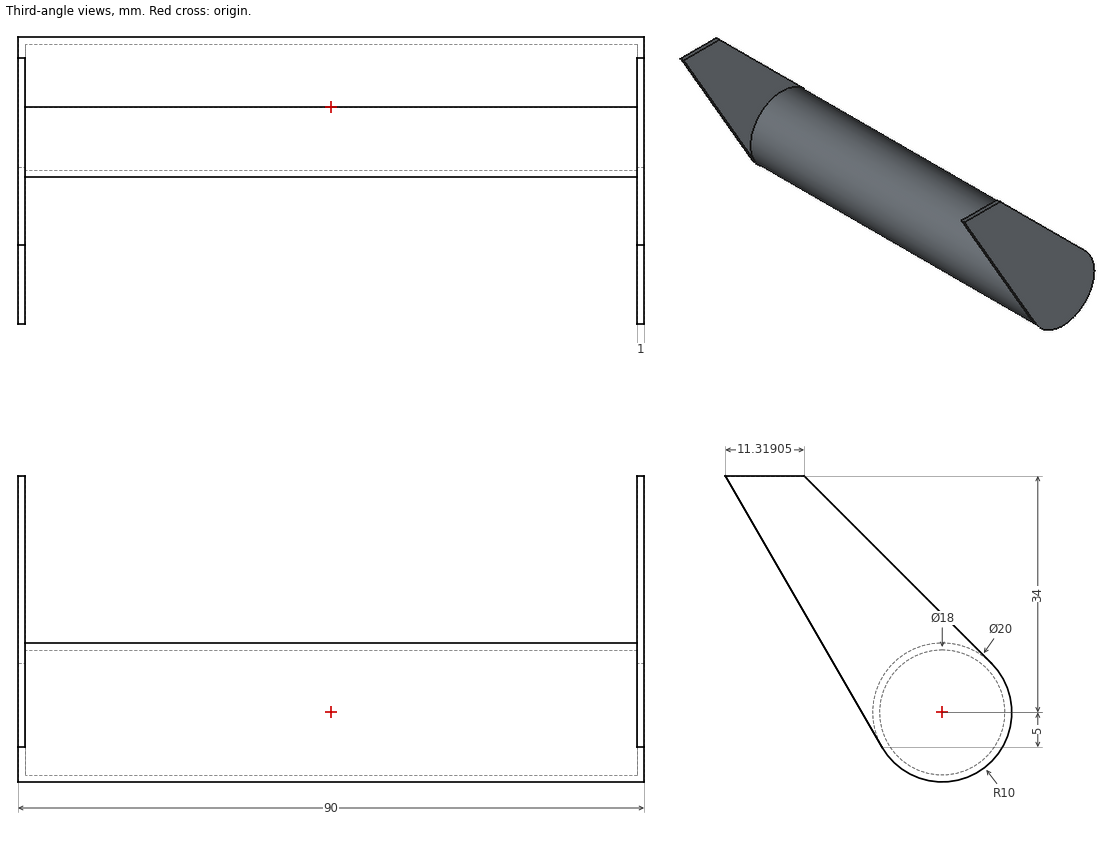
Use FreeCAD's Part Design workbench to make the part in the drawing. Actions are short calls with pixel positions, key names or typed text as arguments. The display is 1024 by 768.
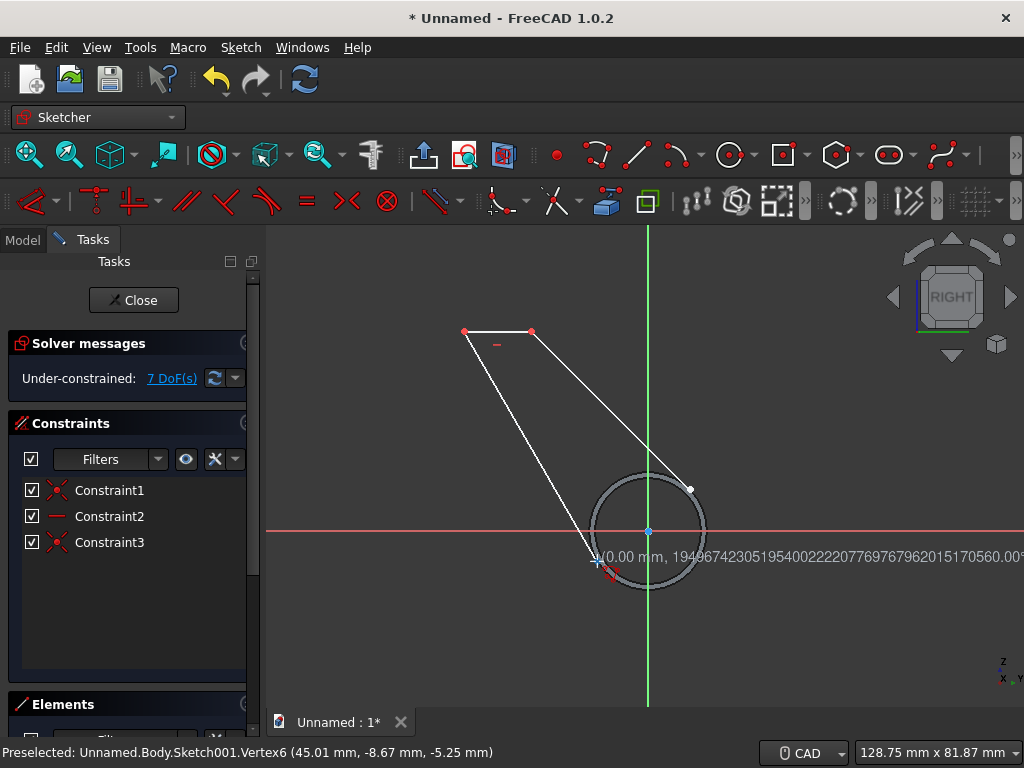
key(g)
key(3)
key(a)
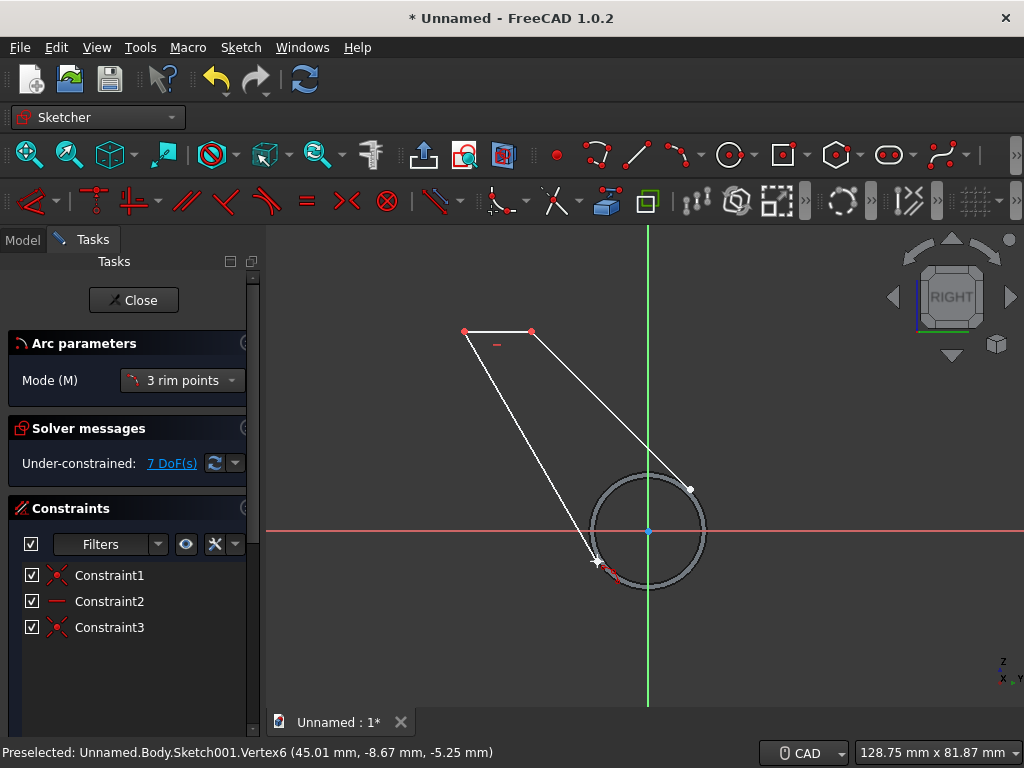
click(597, 562)
click(690, 490)
click(684, 578)
key(Escape)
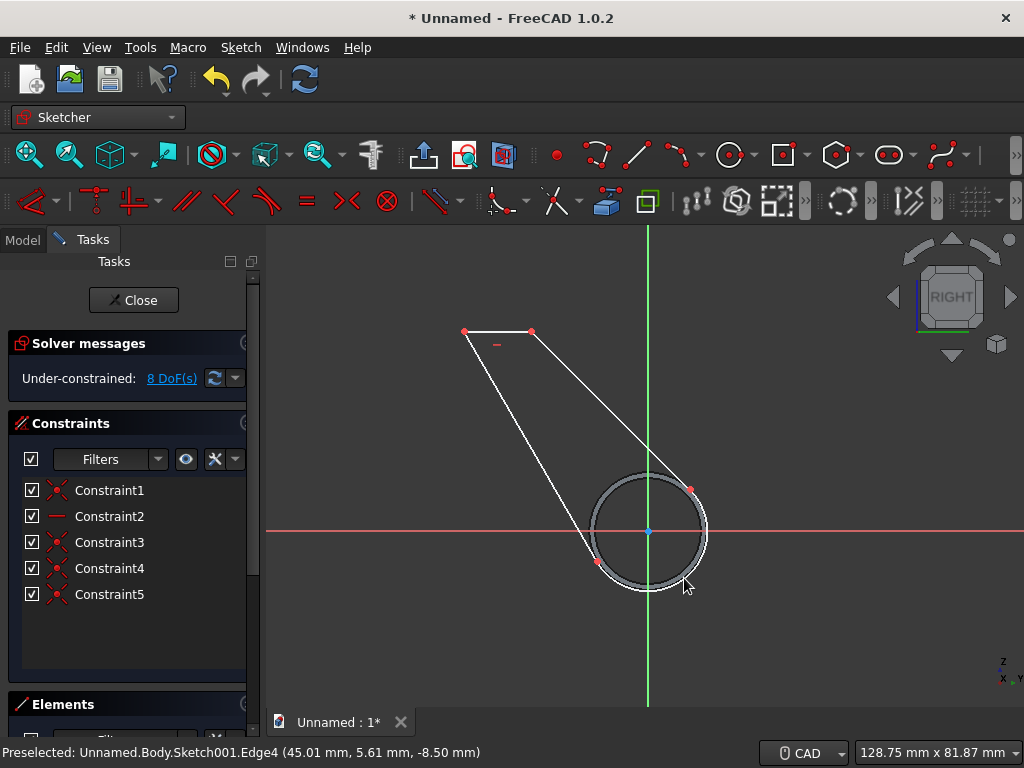
click(579, 379)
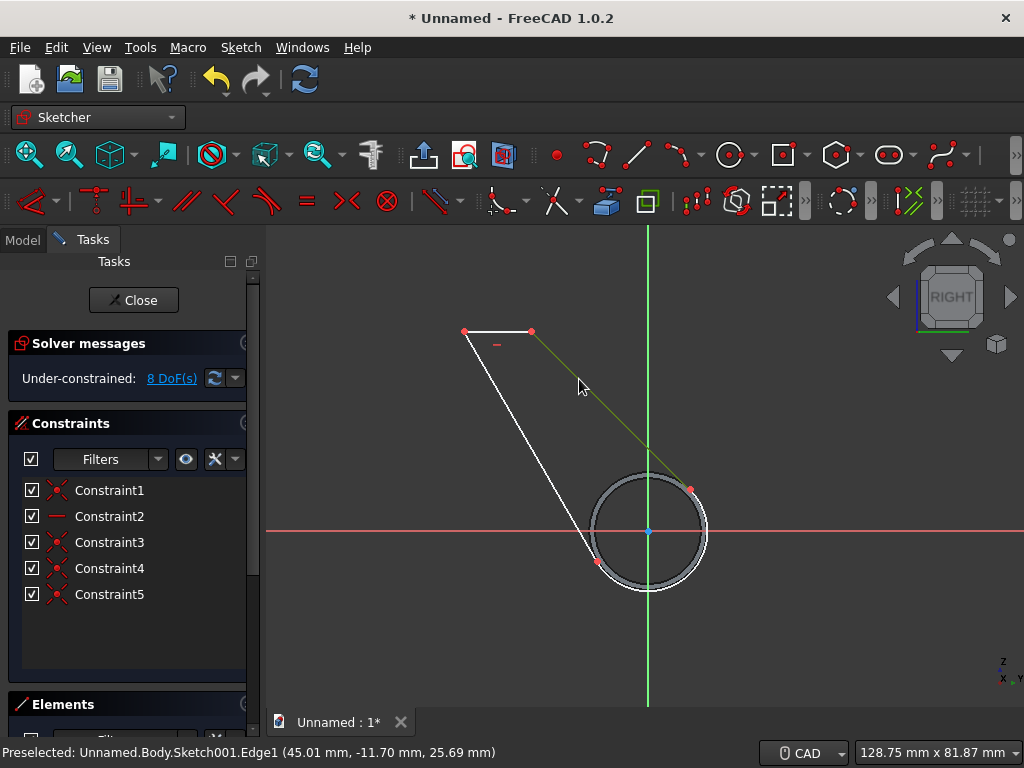
click(647, 591)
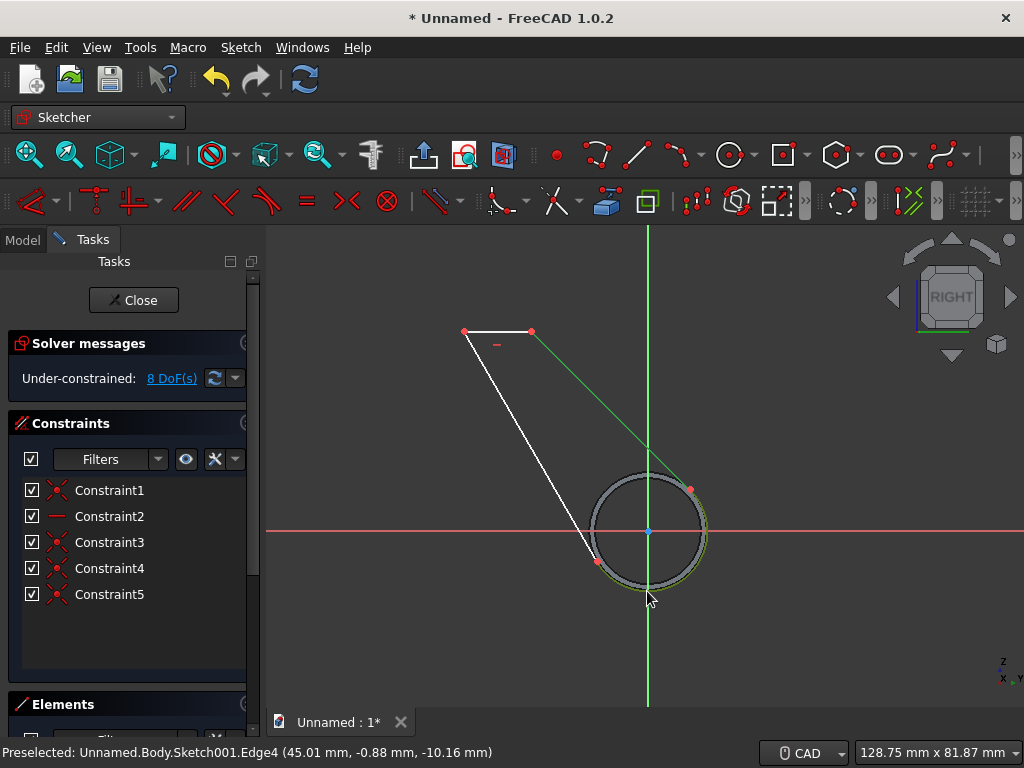
click(268, 202)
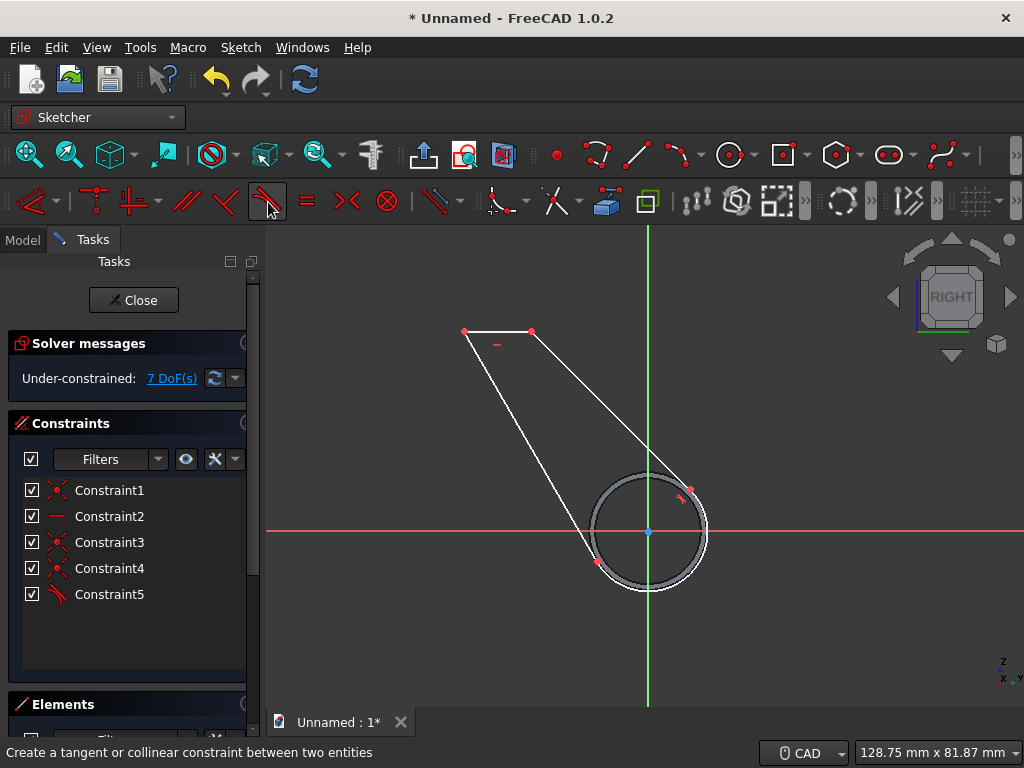
click(504, 401)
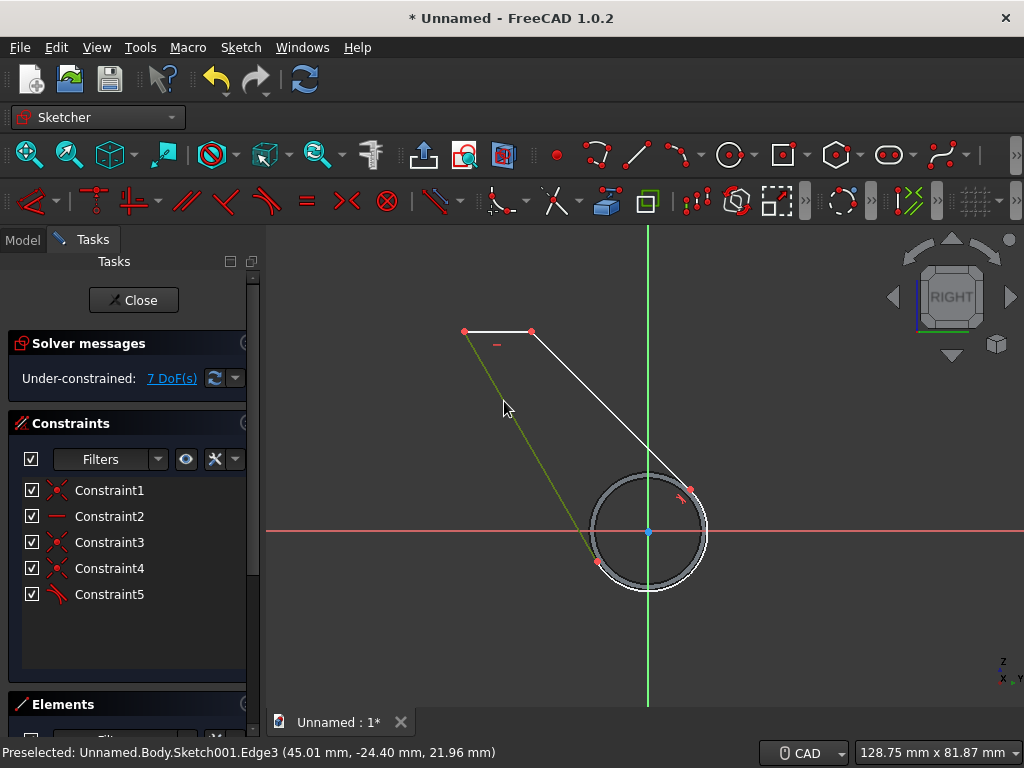
click(647, 591)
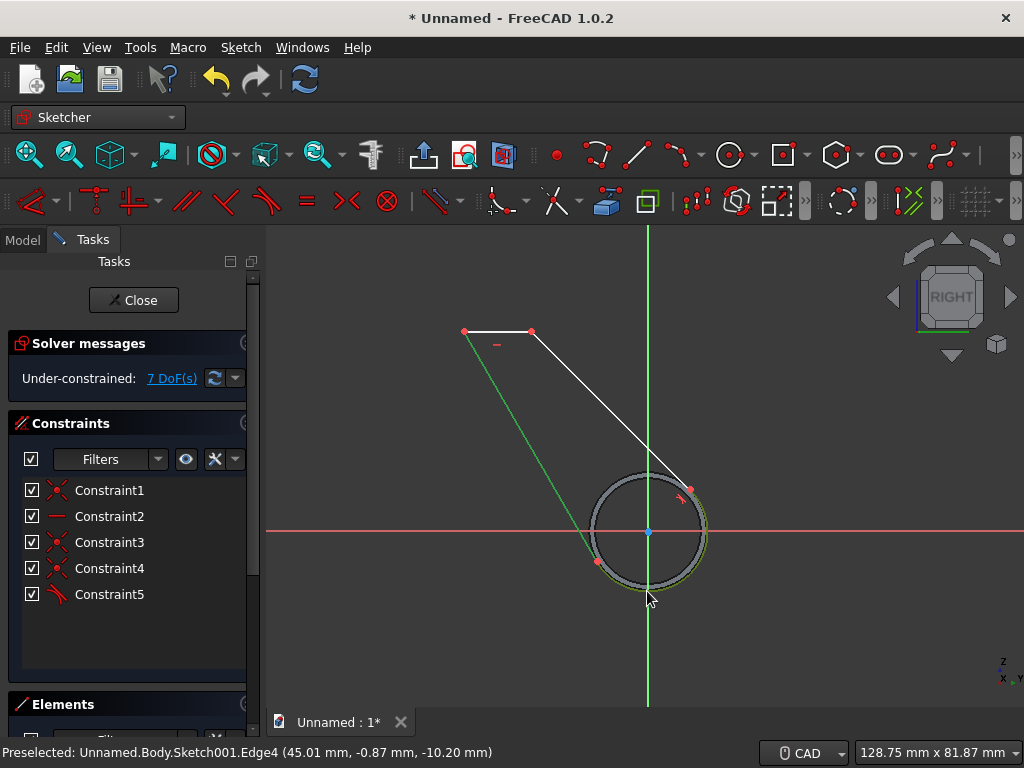
key(t)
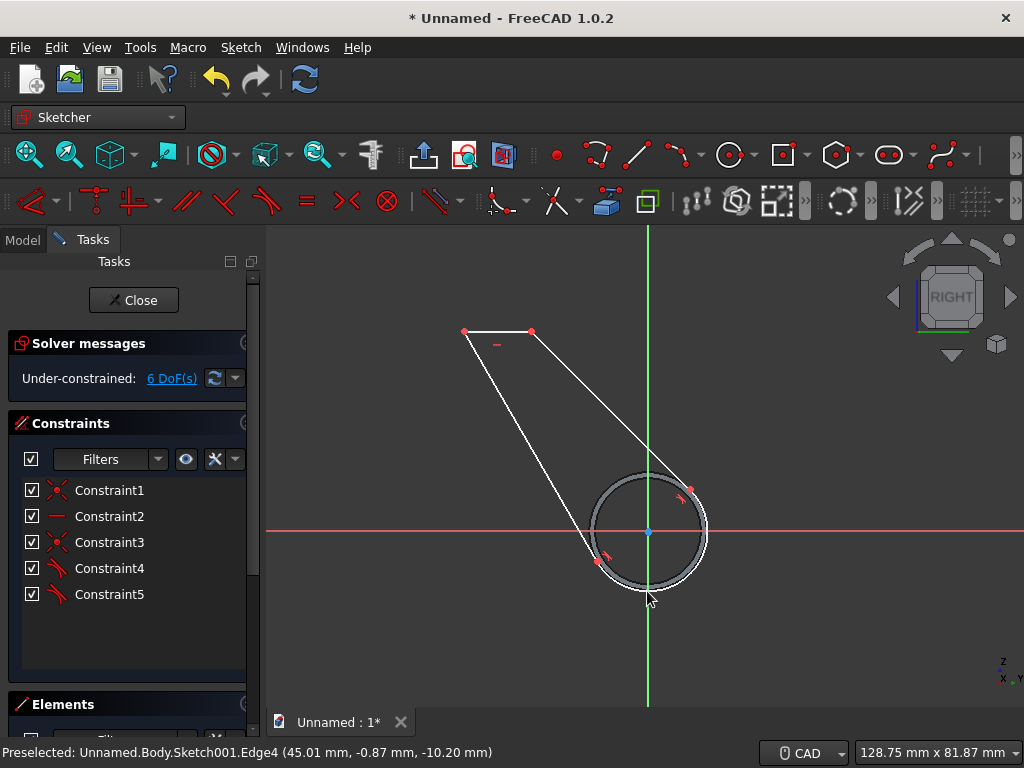
drag(638, 521, 658, 542)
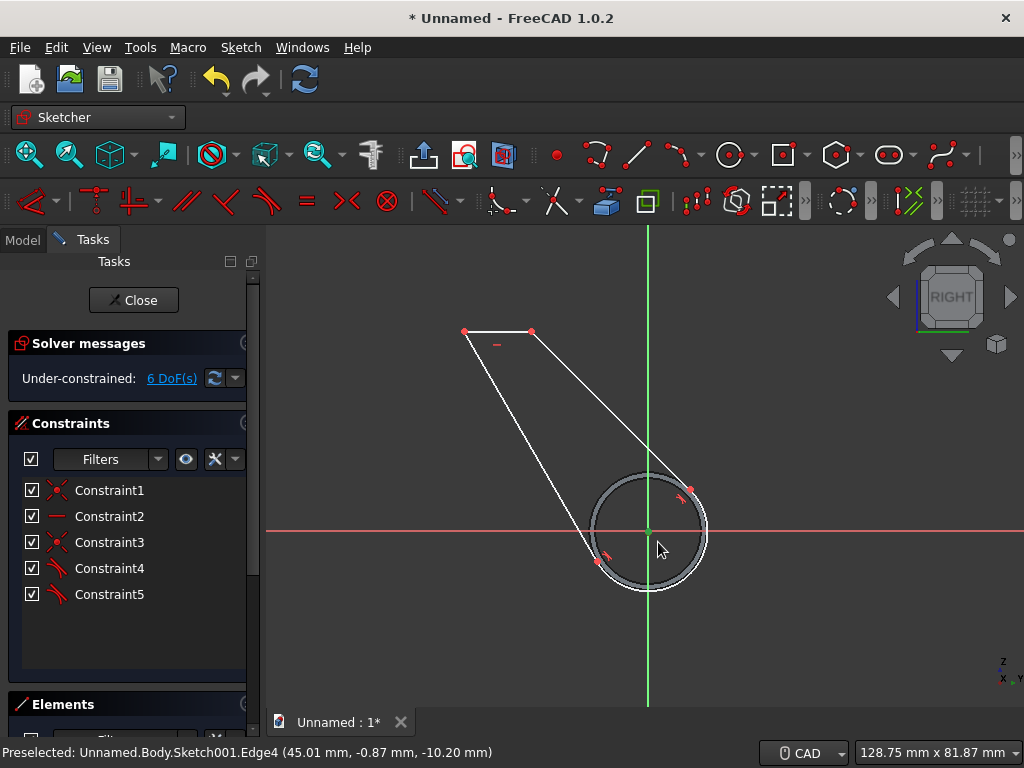
click(94, 202)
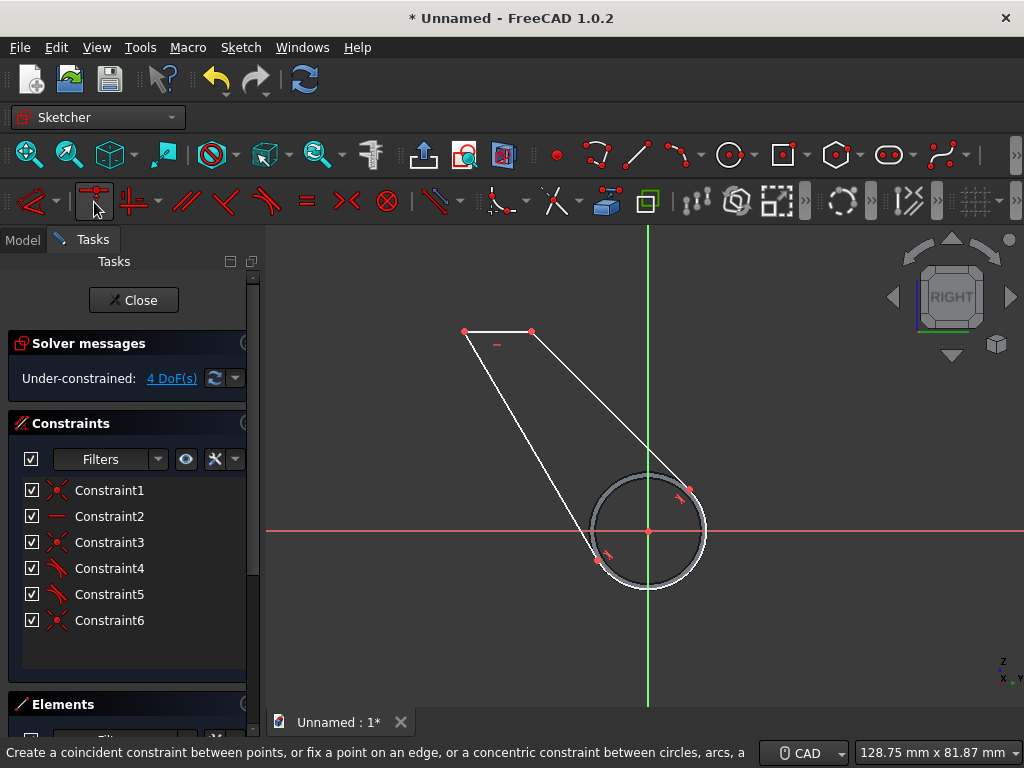
click(32, 202)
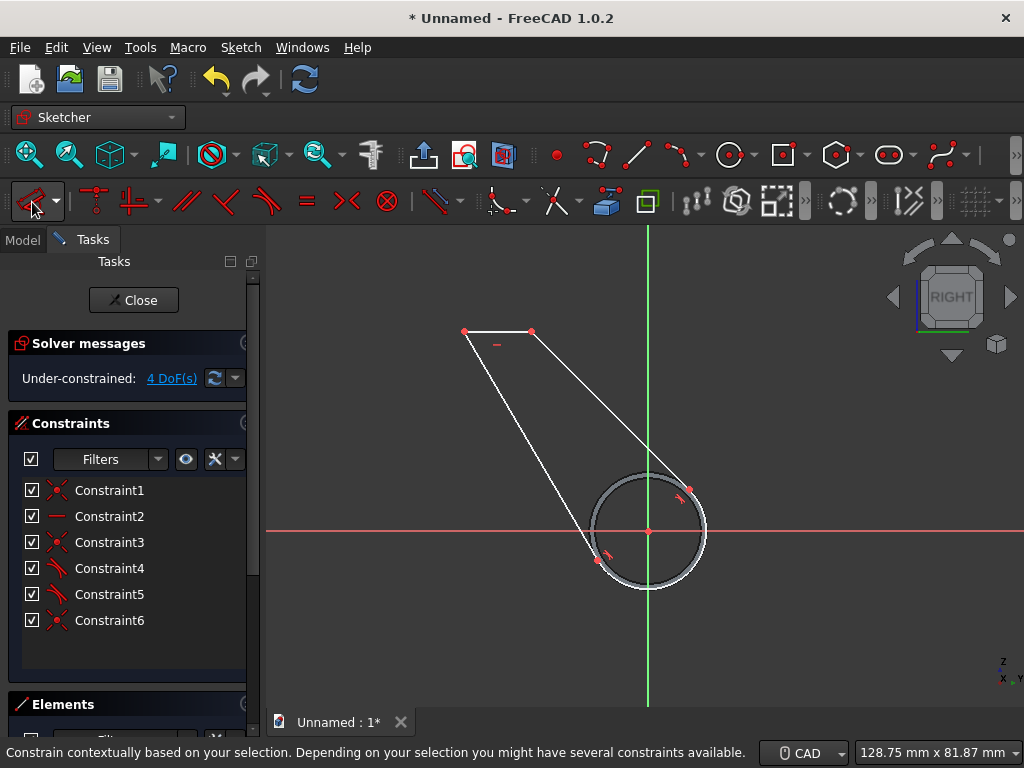
click(647, 589)
click(604, 609)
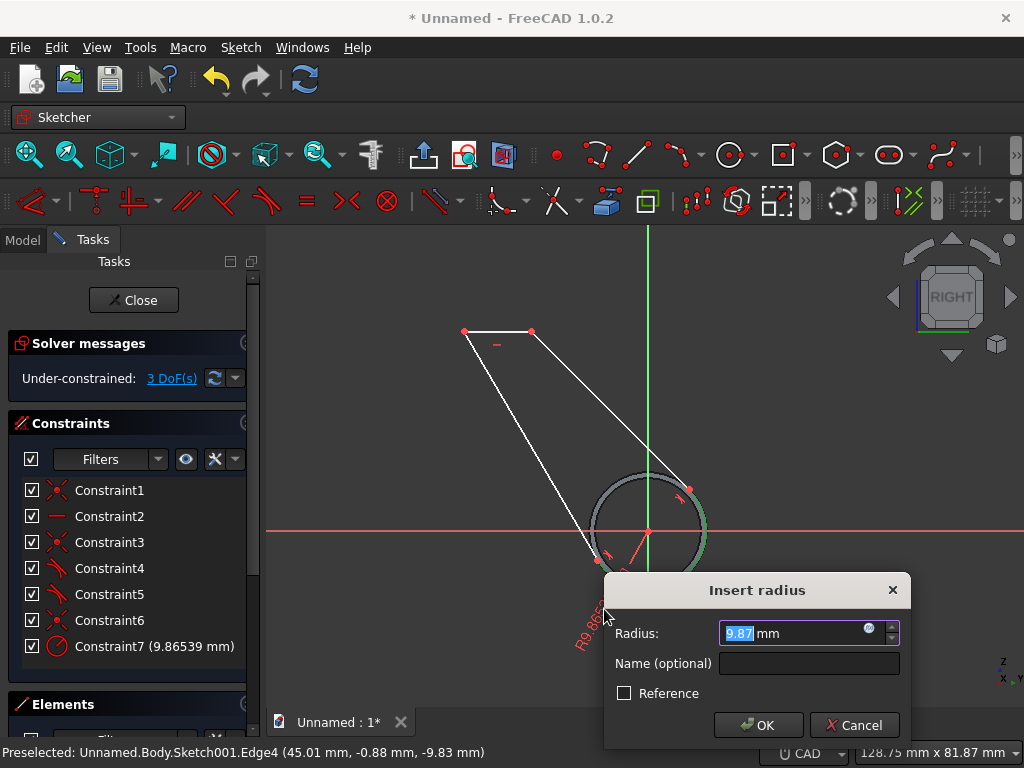
text(10)
key(Return)